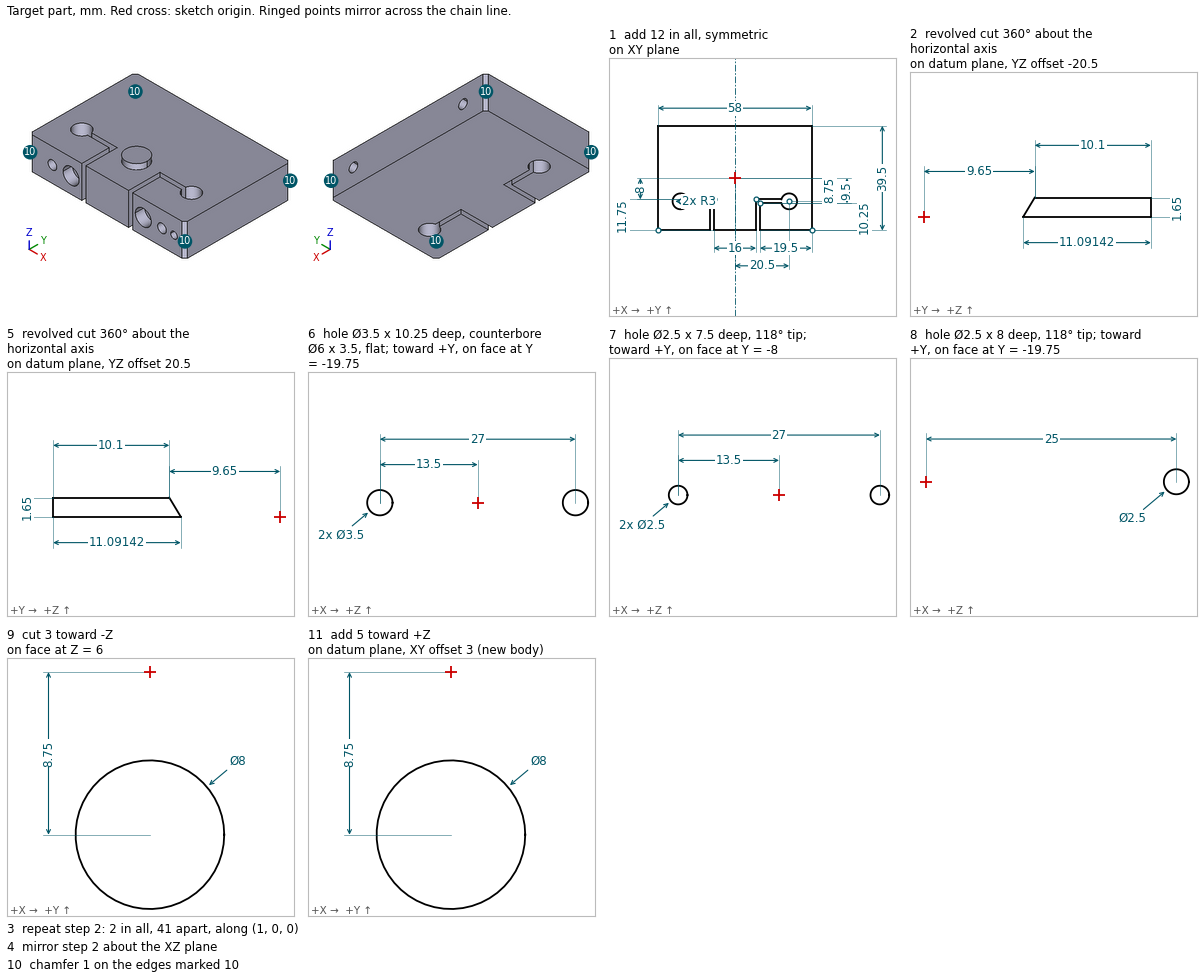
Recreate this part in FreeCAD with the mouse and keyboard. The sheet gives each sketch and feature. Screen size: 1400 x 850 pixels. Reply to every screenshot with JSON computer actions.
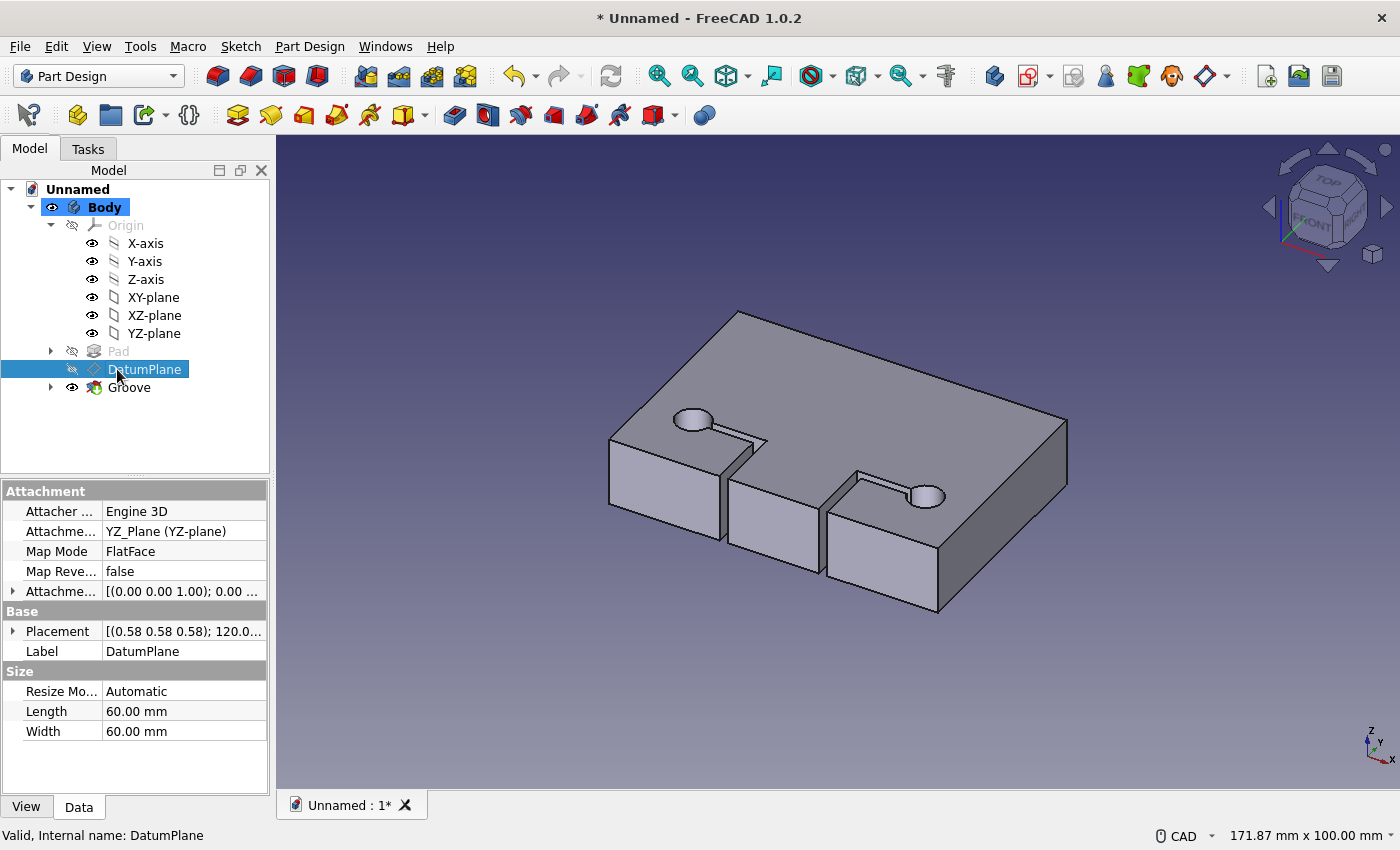
{"action": "left_click", "coordinate": [117, 387]}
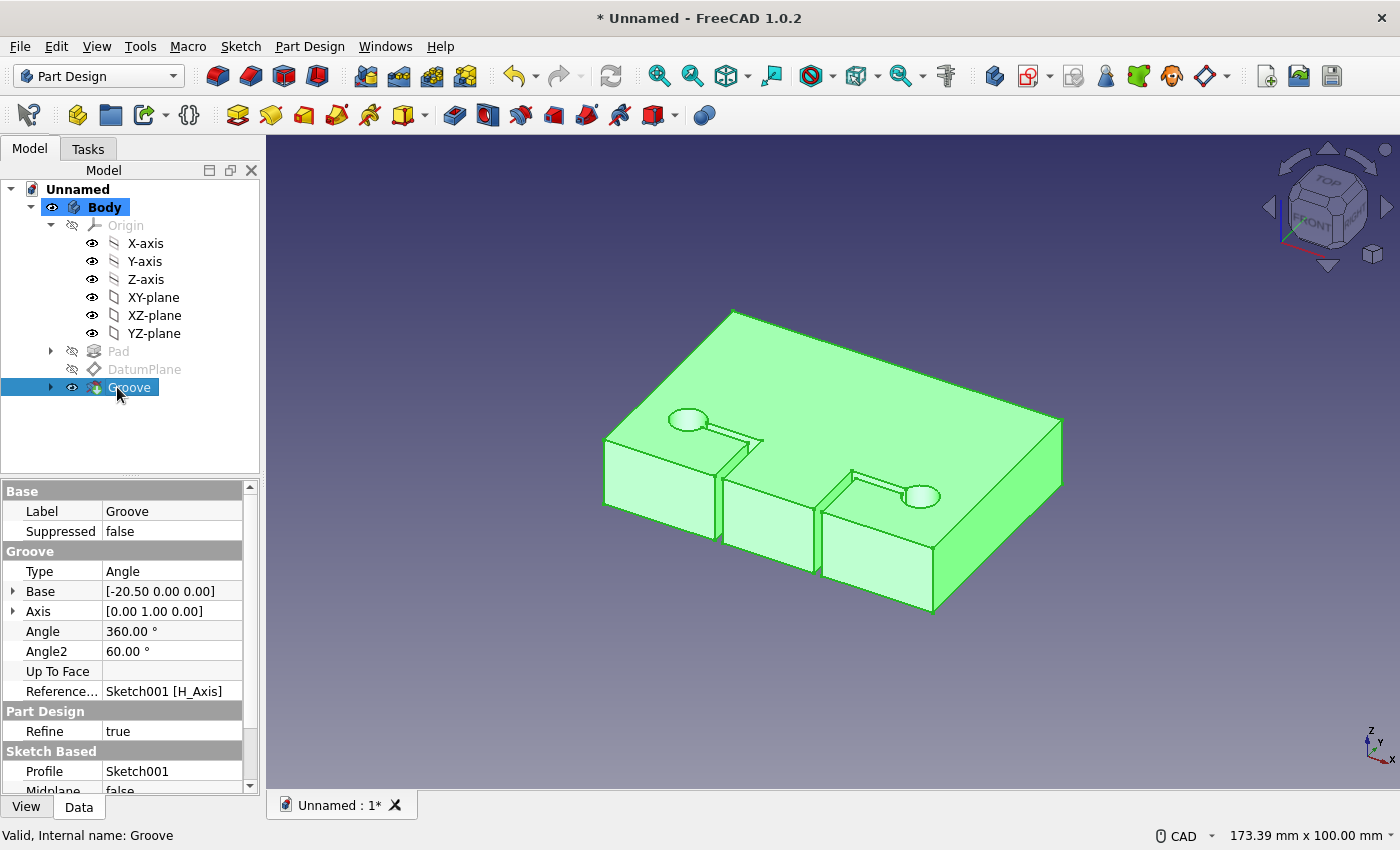
{"action": "left_click", "coordinate": [399, 76]}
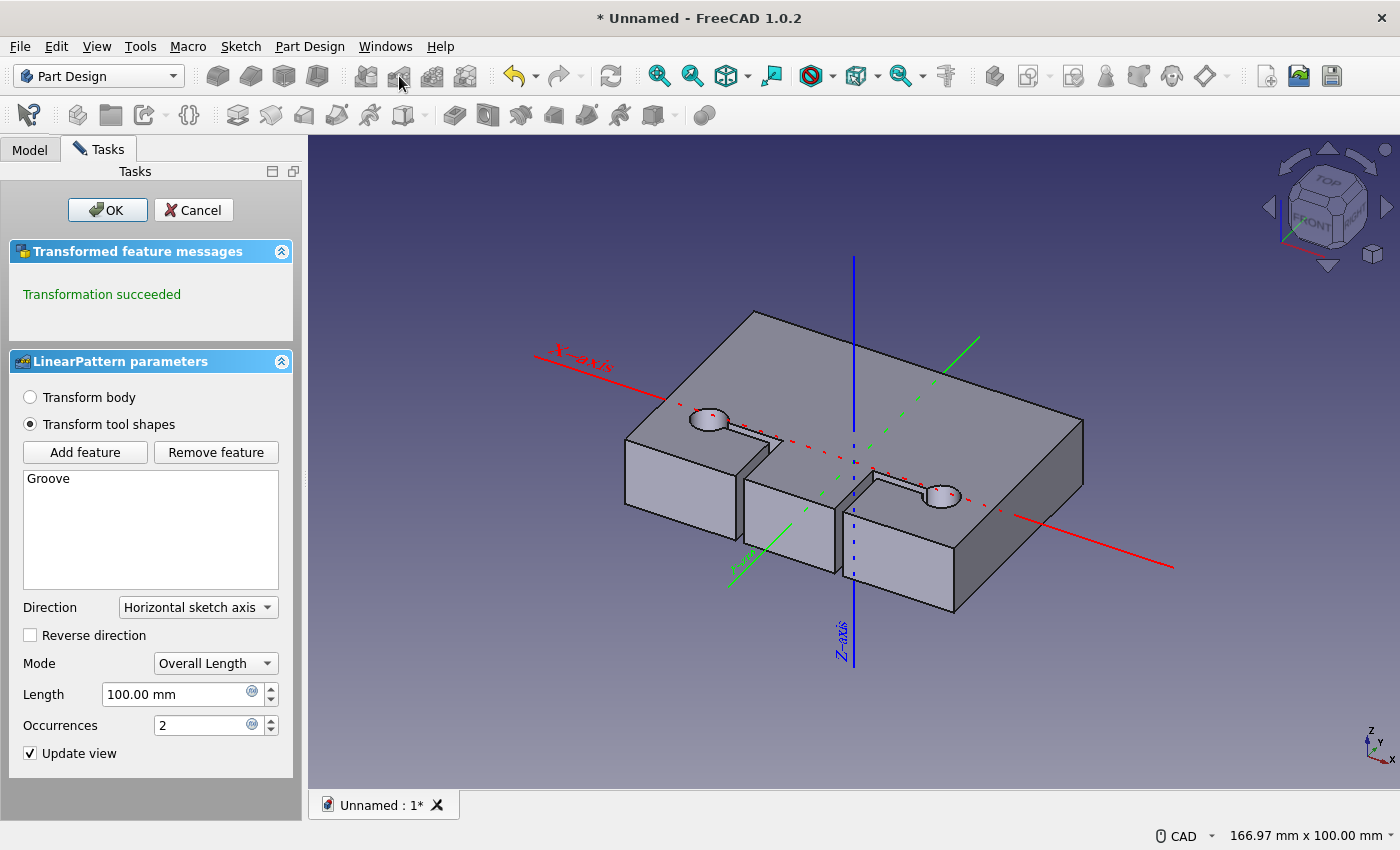
{"action": "left_click", "coordinate": [199, 608]}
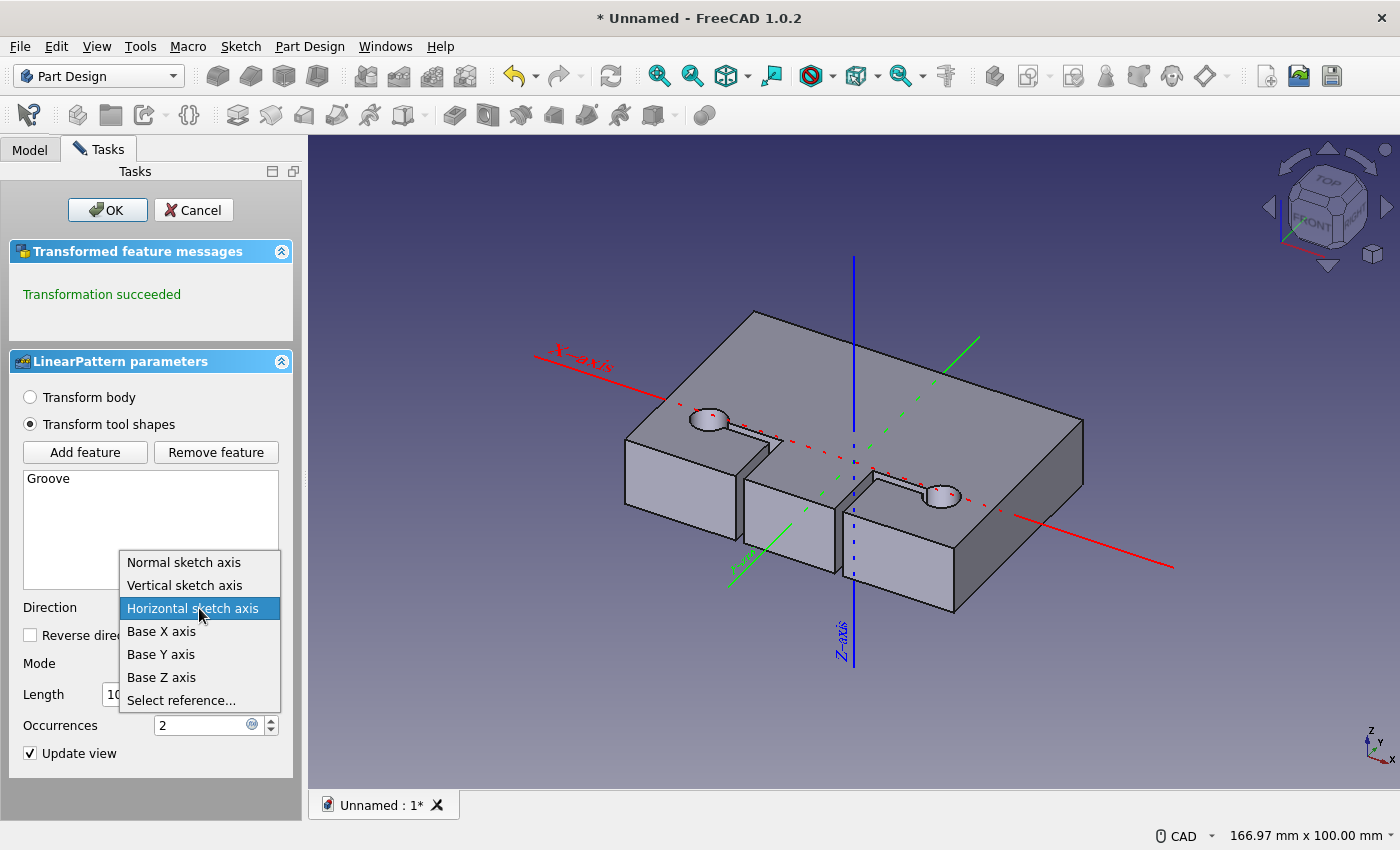
{"action": "left_click", "coordinate": [198, 632]}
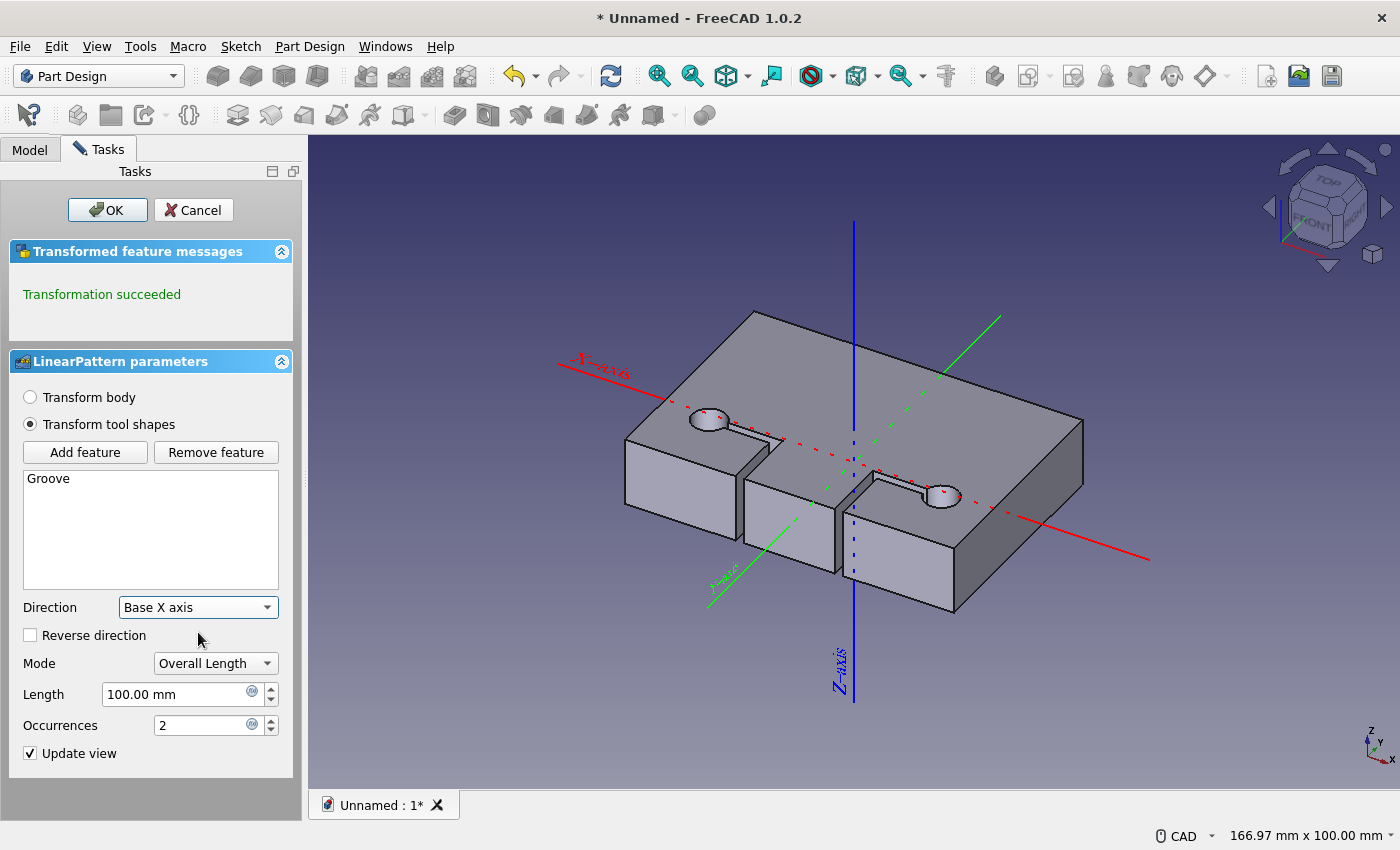
{"action": "left_click", "coordinate": [216, 664]}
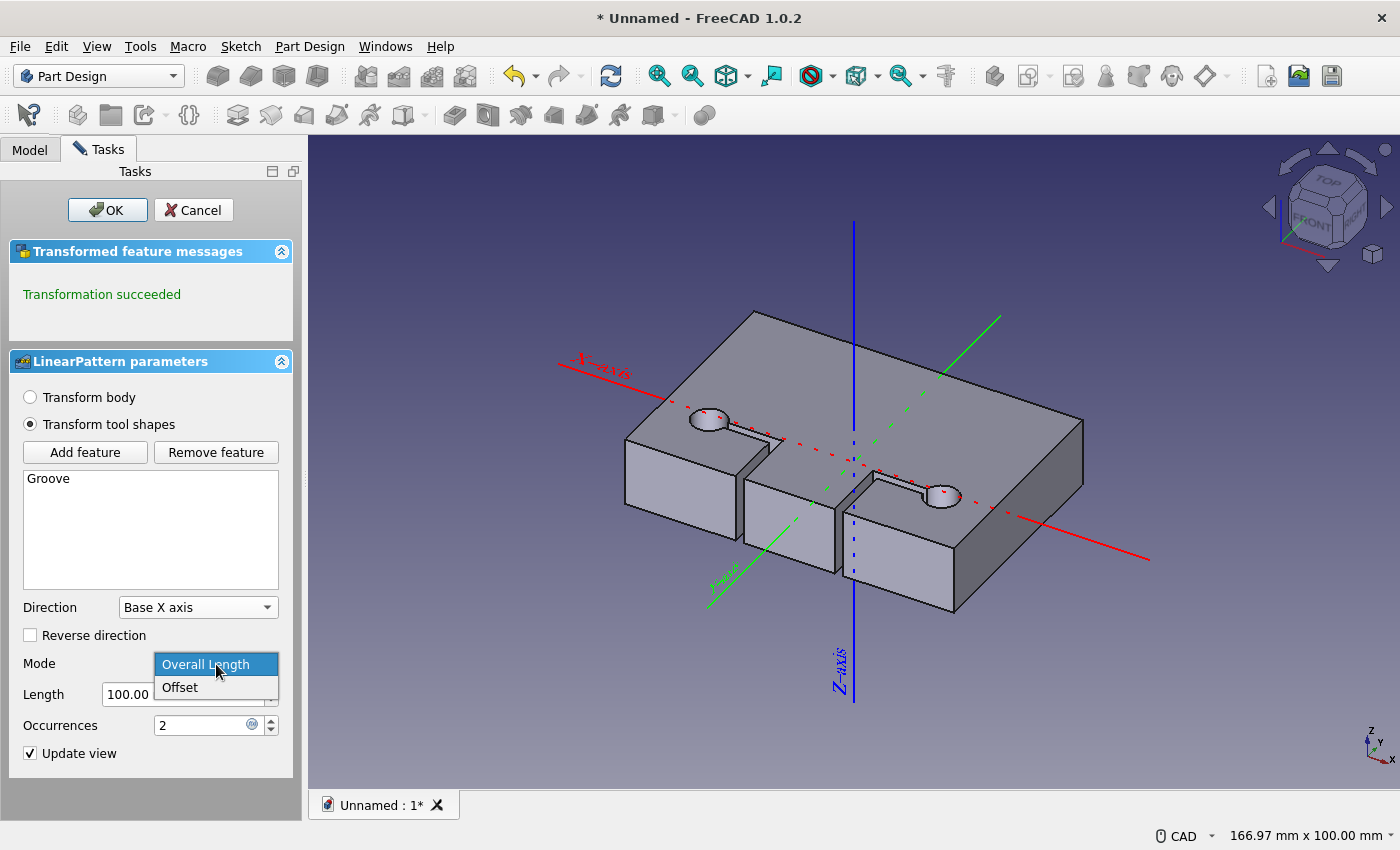
{"action": "left_click", "coordinate": [214, 688]}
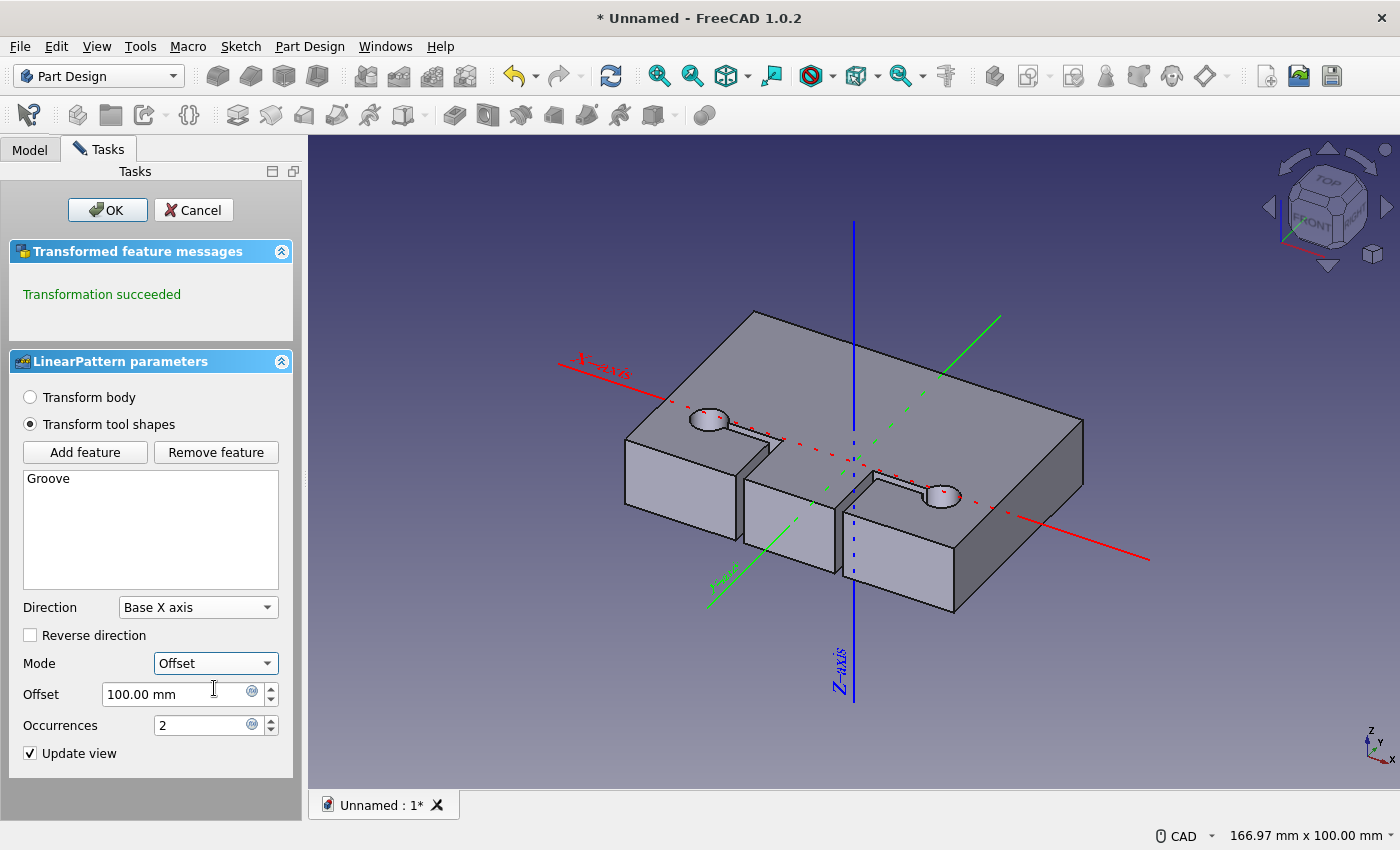
{"action": "triple_click", "coordinate": [184, 694]}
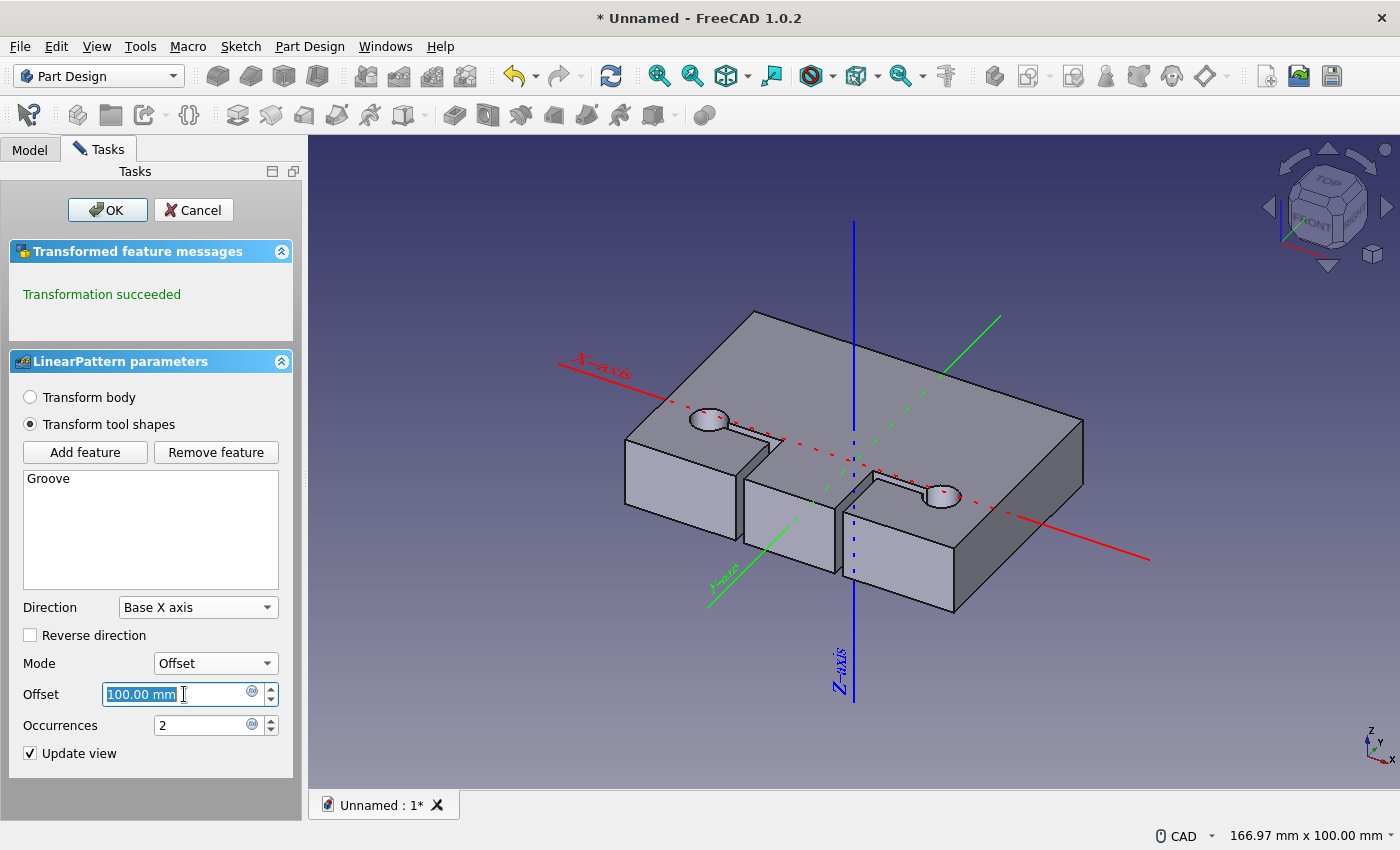
{"action": "type", "text": "41"}
{"action": "key", "text": "Tab"}